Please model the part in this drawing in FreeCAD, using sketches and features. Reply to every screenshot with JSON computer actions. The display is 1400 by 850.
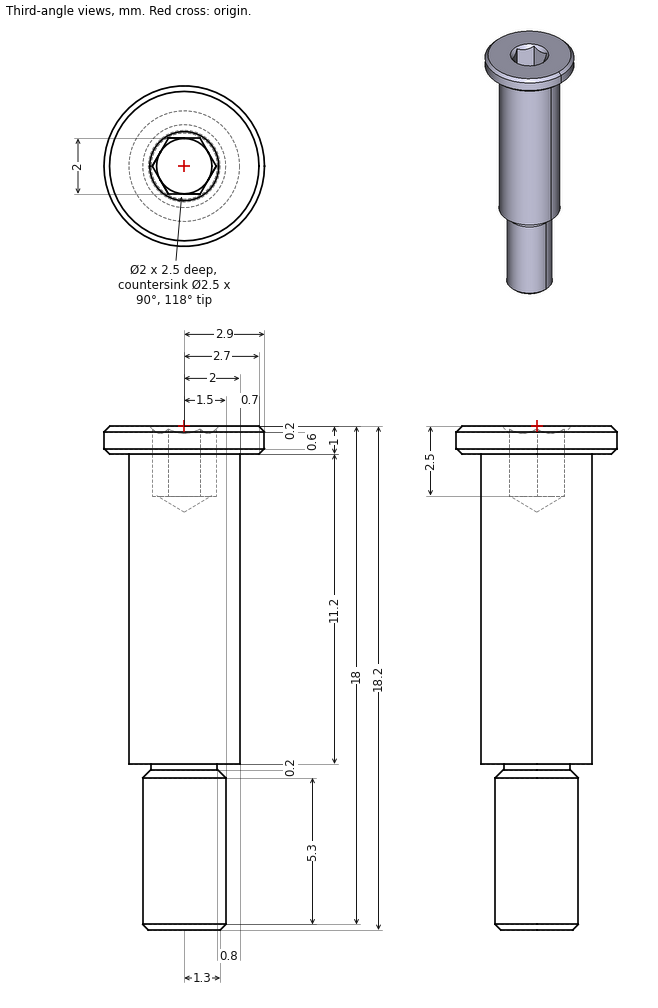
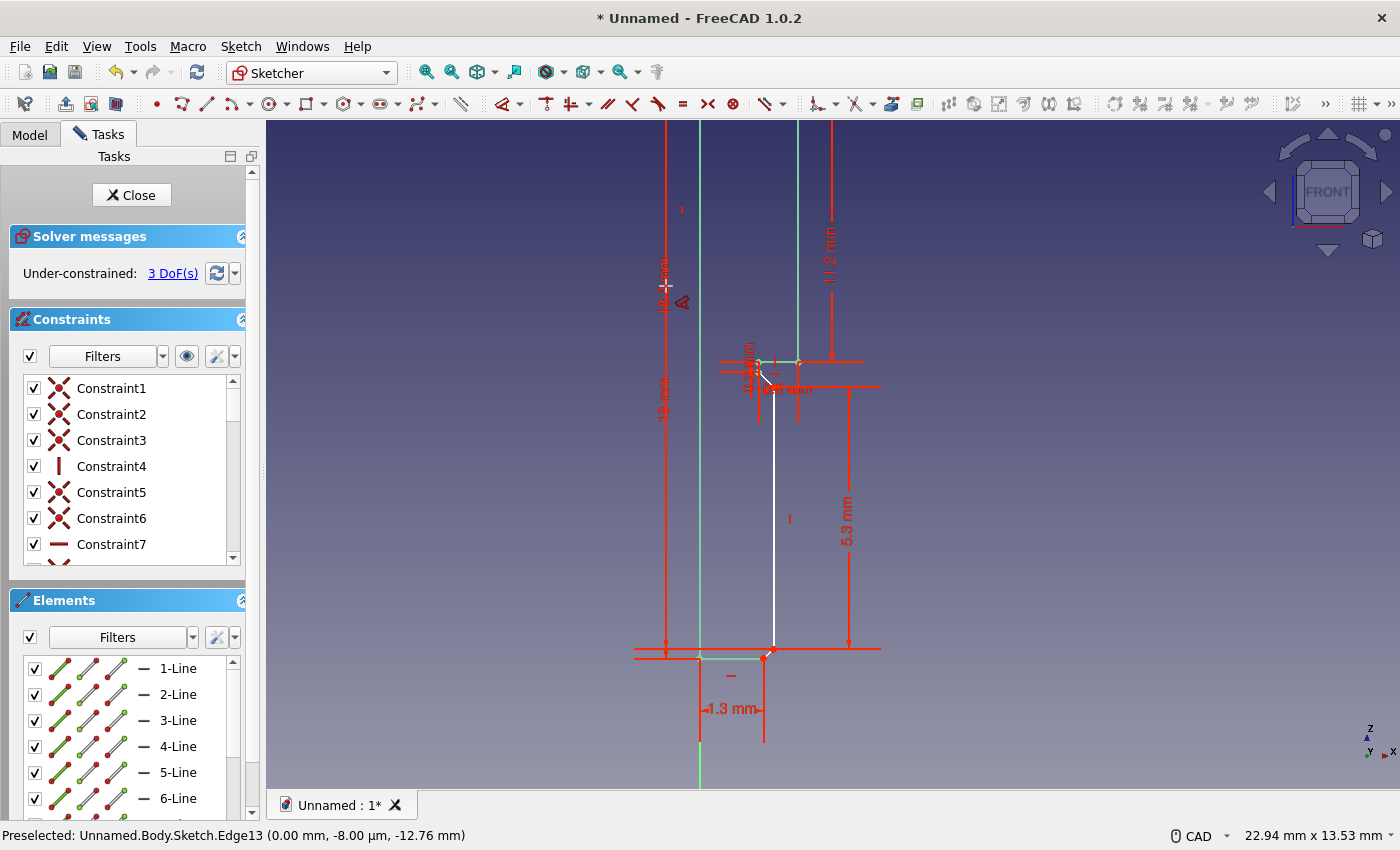
{"action": "scroll", "coordinate": [759, 655], "scroll_direction": "down", "scroll_amount": 4}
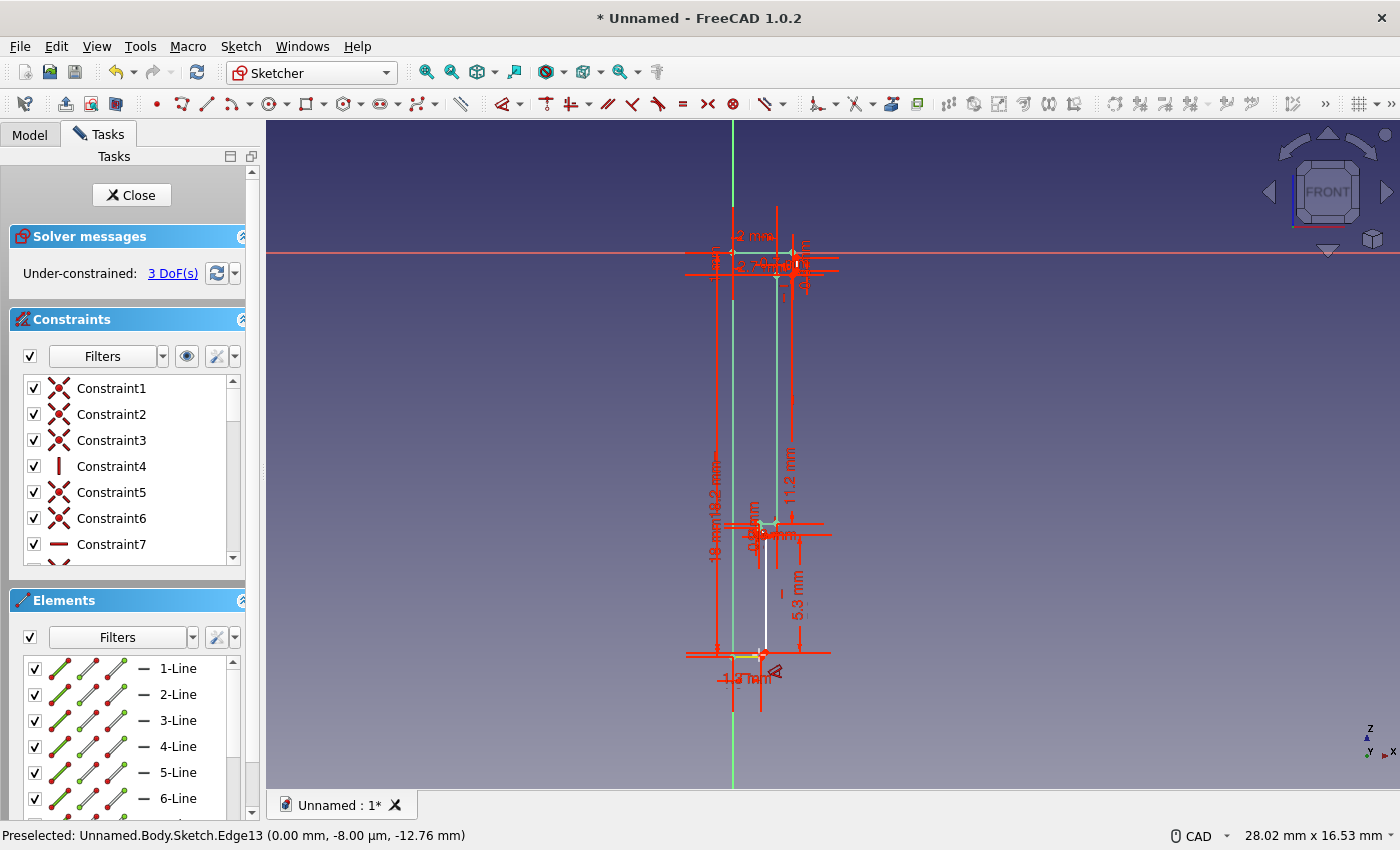
{"action": "scroll", "coordinate": [797, 258], "scroll_direction": "up", "scroll_amount": 4}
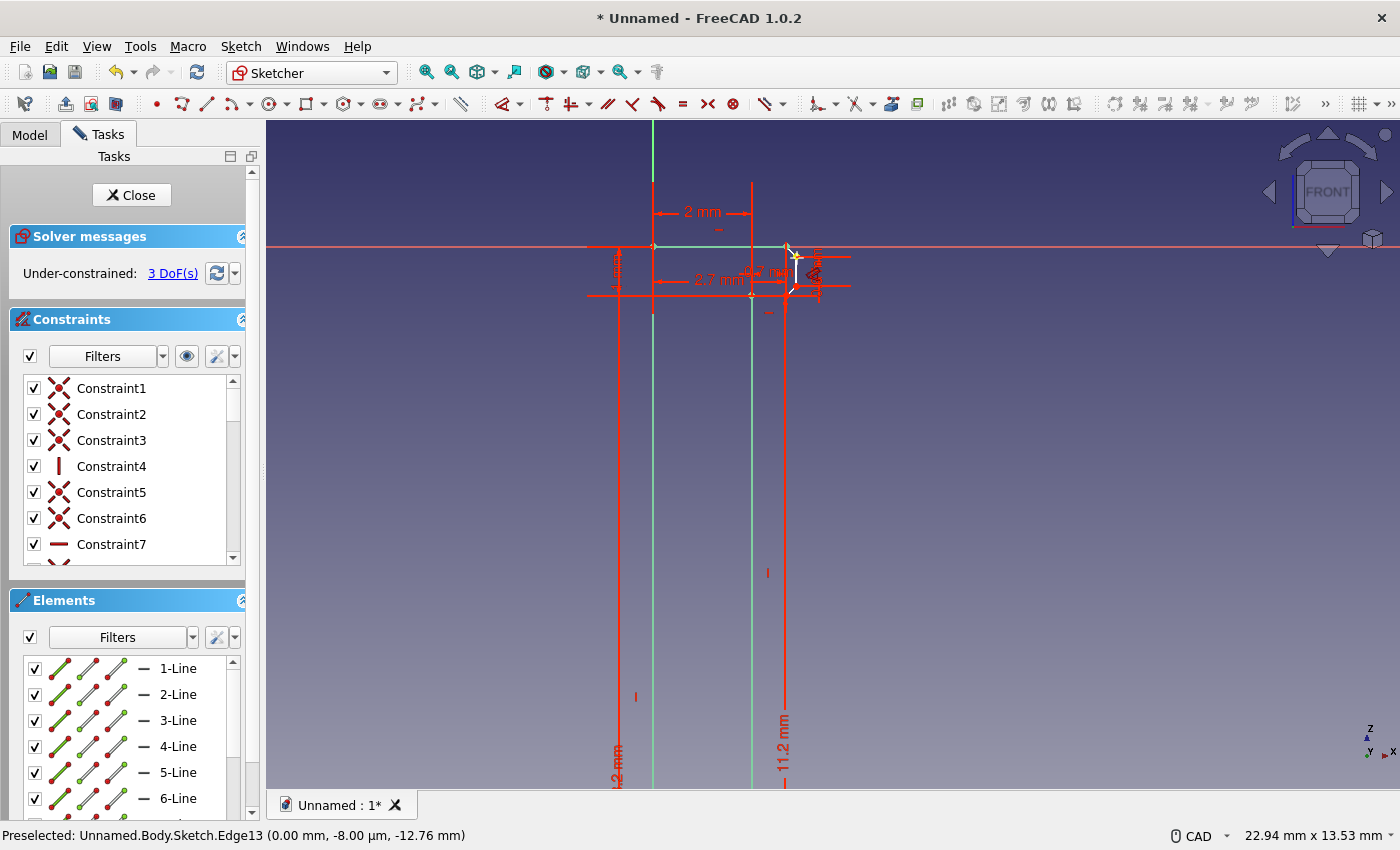
{"action": "left_click", "coordinate": [796, 257]}
{"action": "left_click", "coordinate": [775, 212]}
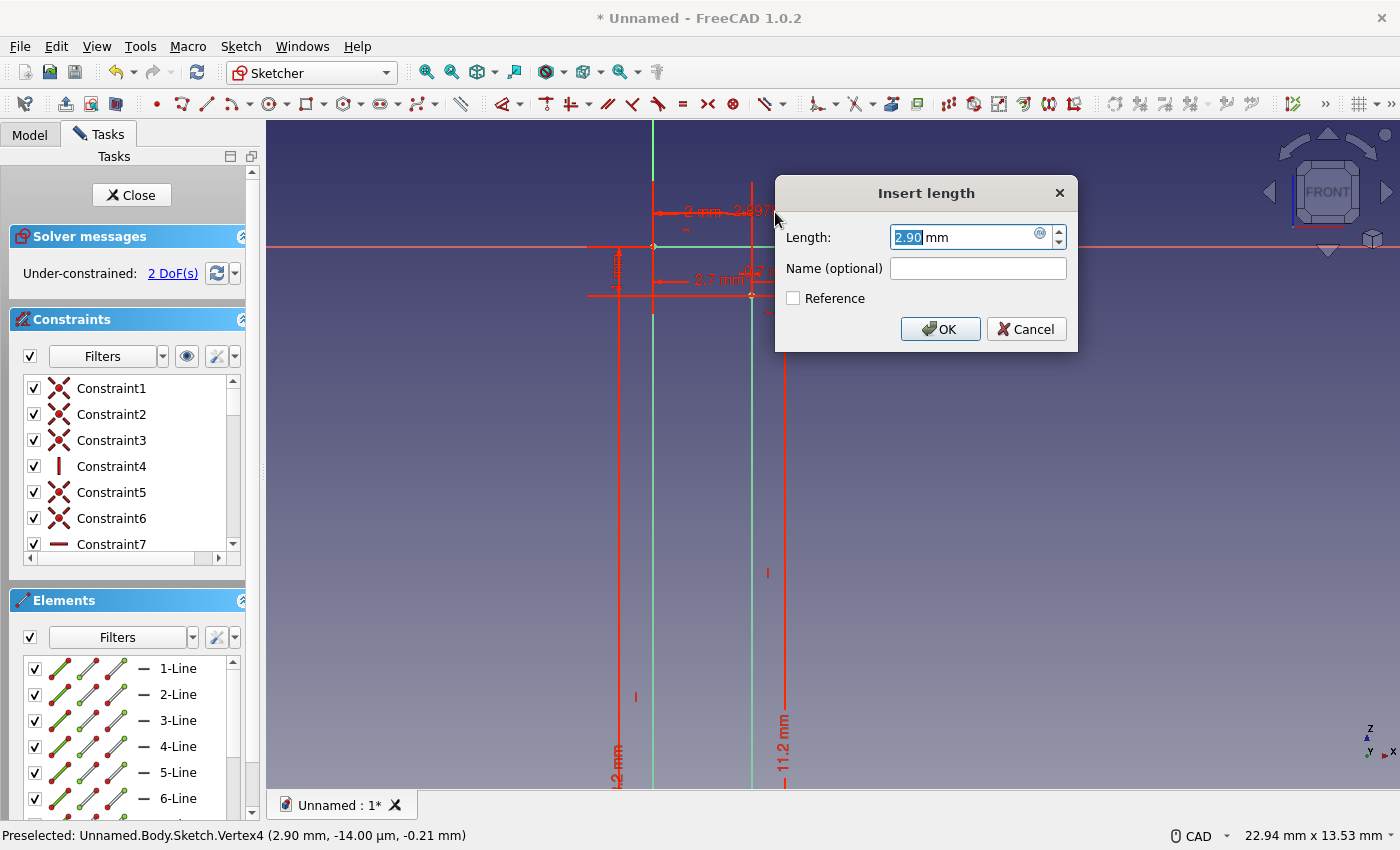
{"action": "type", "text": "2.9"}
{"action": "key", "text": "Return"}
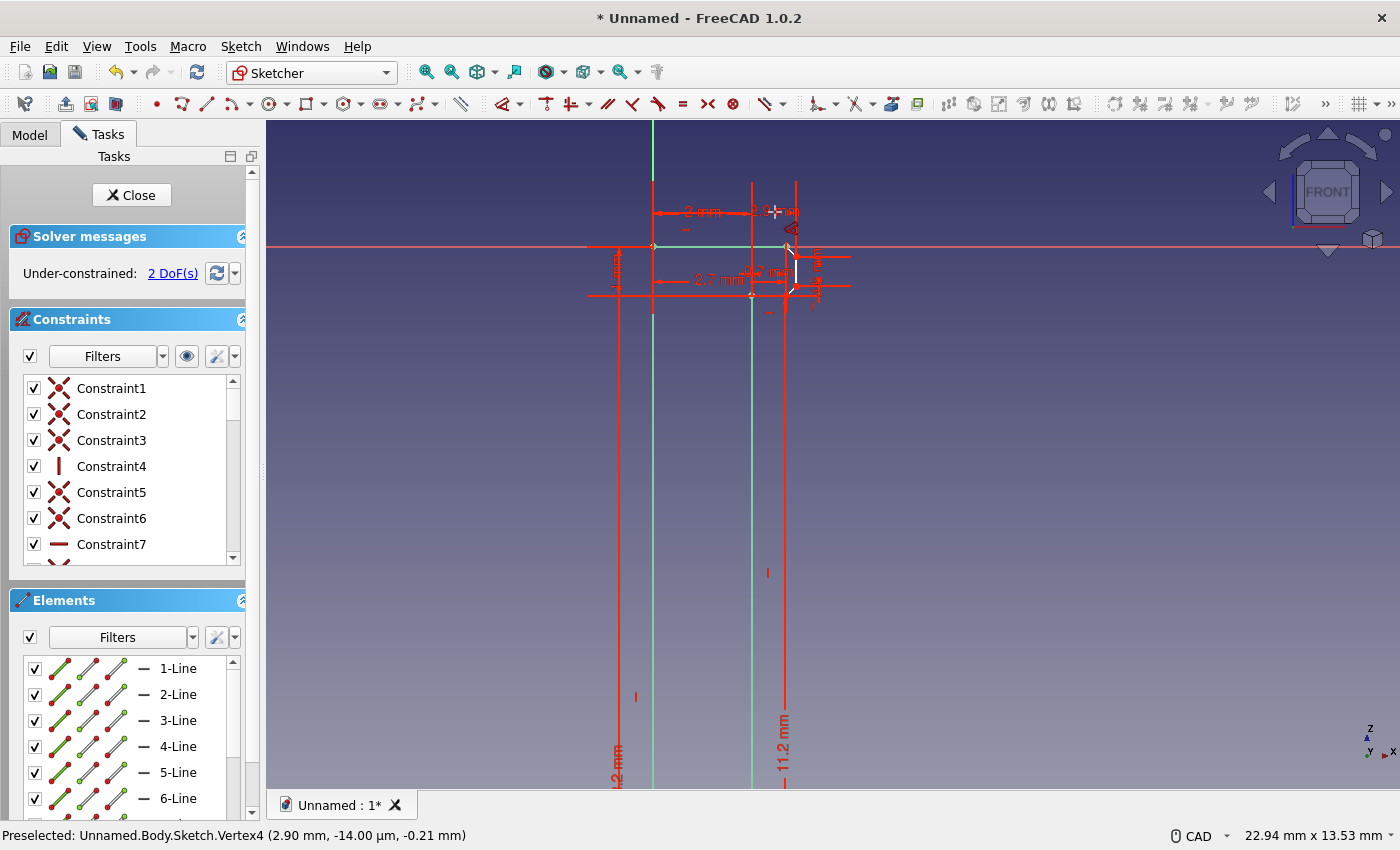
{"action": "scroll", "coordinate": [796, 257], "scroll_direction": "up", "scroll_amount": 7}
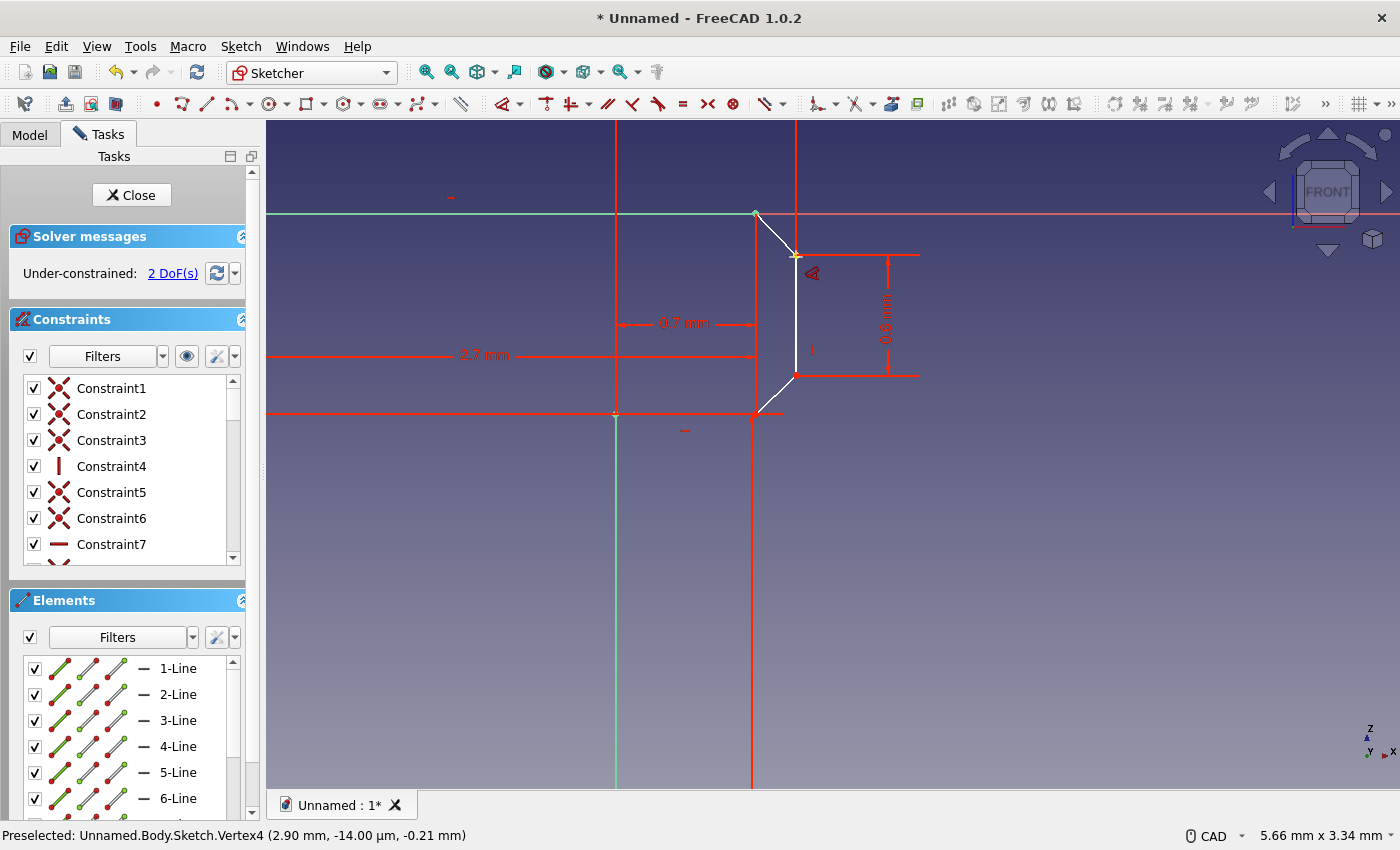
{"action": "left_click", "coordinate": [796, 255]}
{"action": "left_click", "coordinate": [830, 235]}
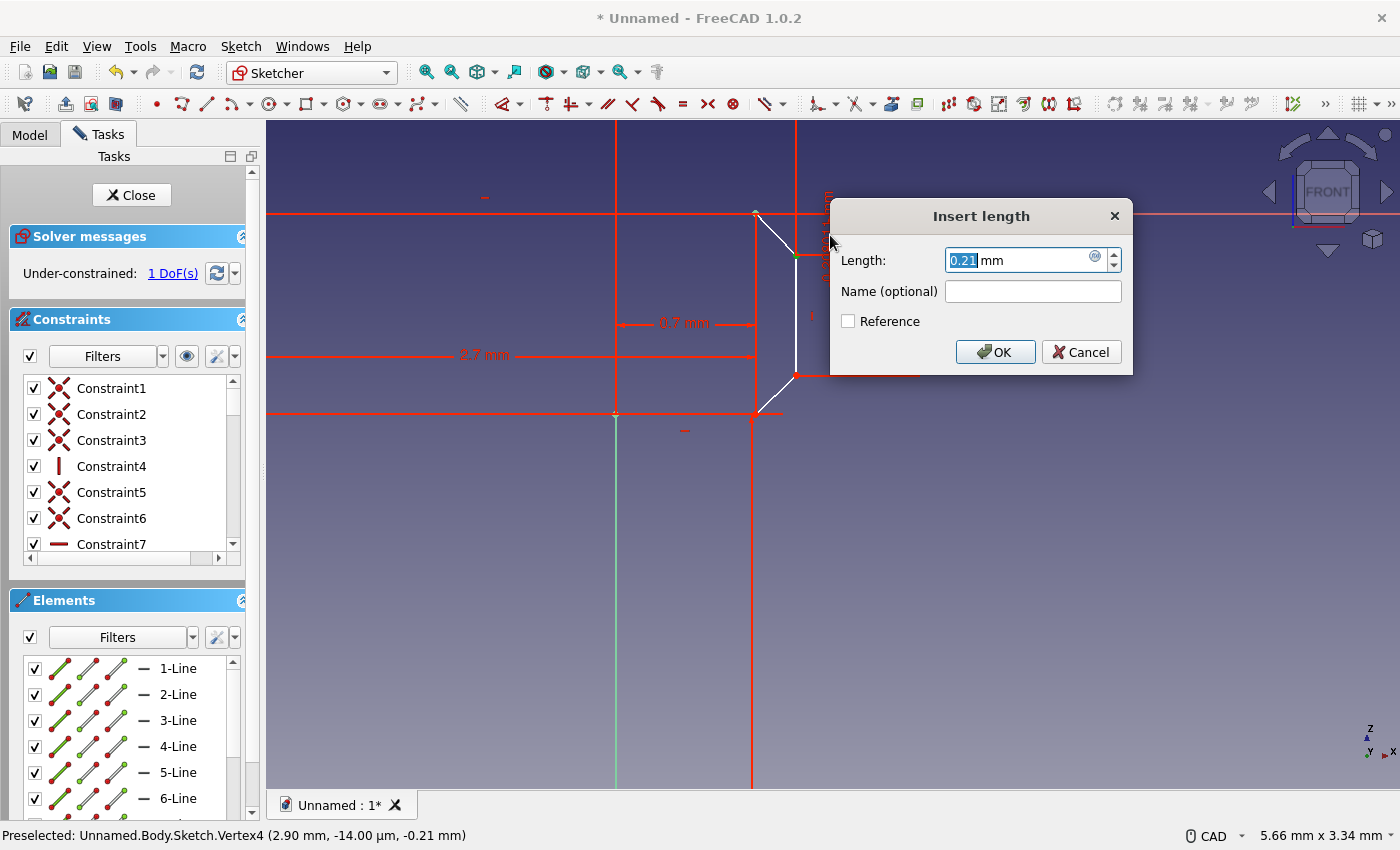
{"action": "type", "text": "0.2"}
{"action": "key", "text": "Return"}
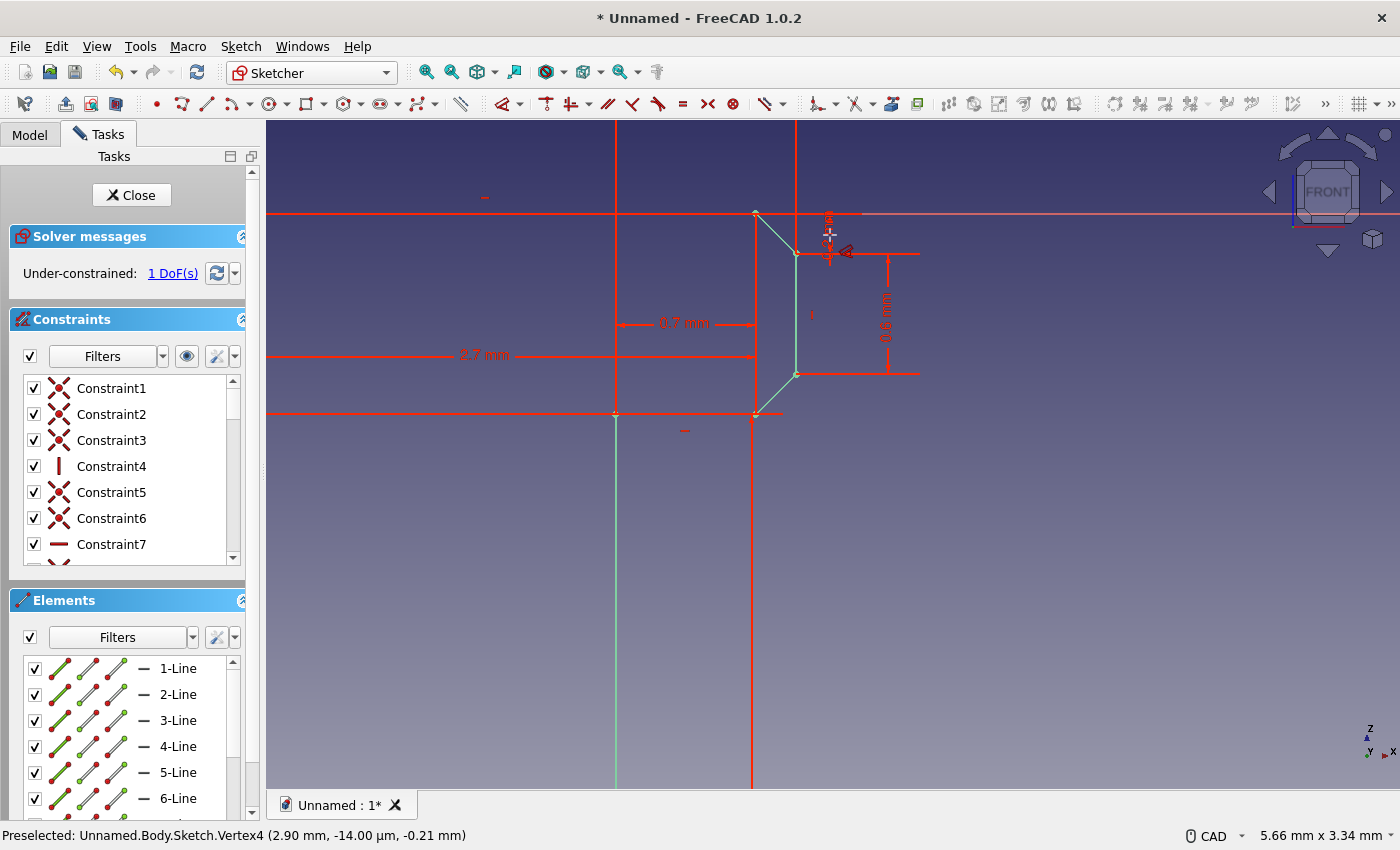
{"action": "scroll", "coordinate": [797, 257], "scroll_direction": "down", "scroll_amount": 11}